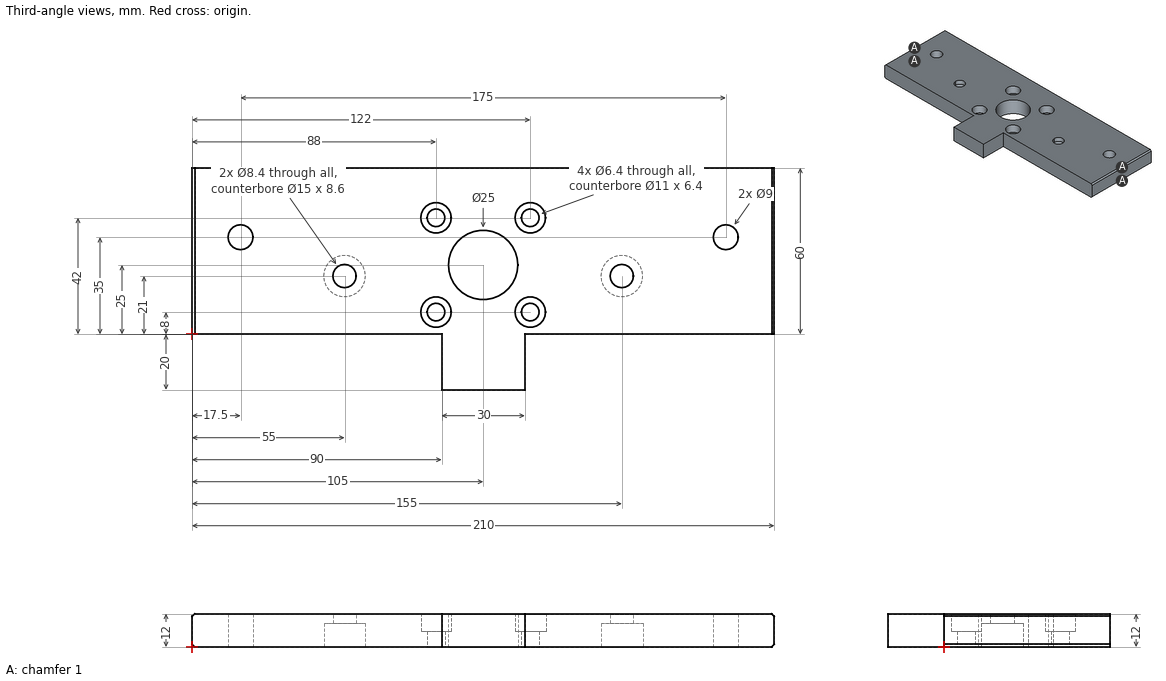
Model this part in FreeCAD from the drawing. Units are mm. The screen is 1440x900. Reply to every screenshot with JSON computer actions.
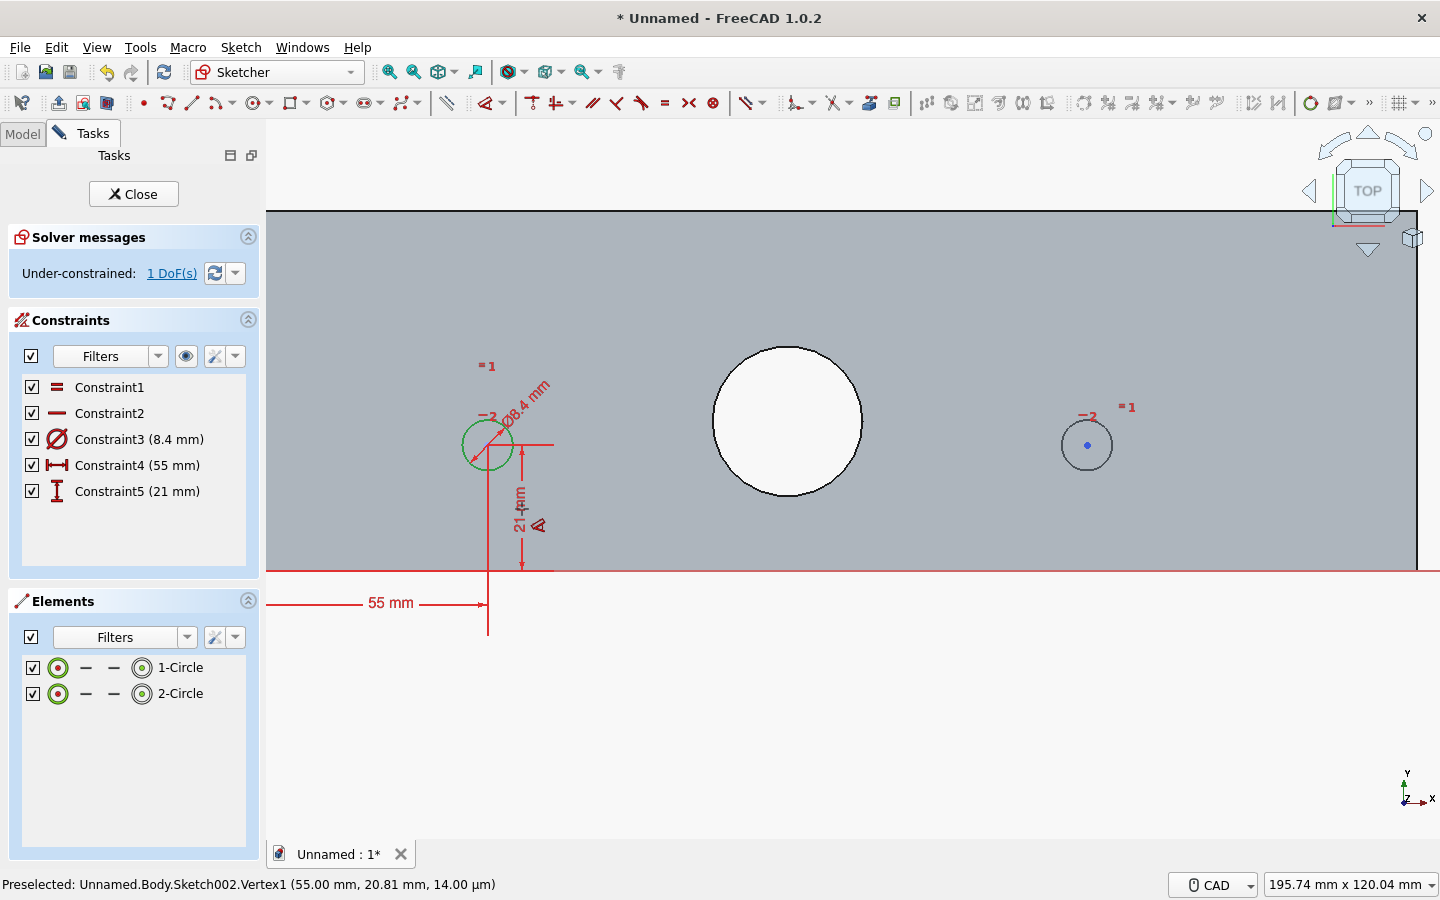
{"action": "left_click", "coordinate": [1087, 445]}
{"action": "left_click", "coordinate": [691, 605]}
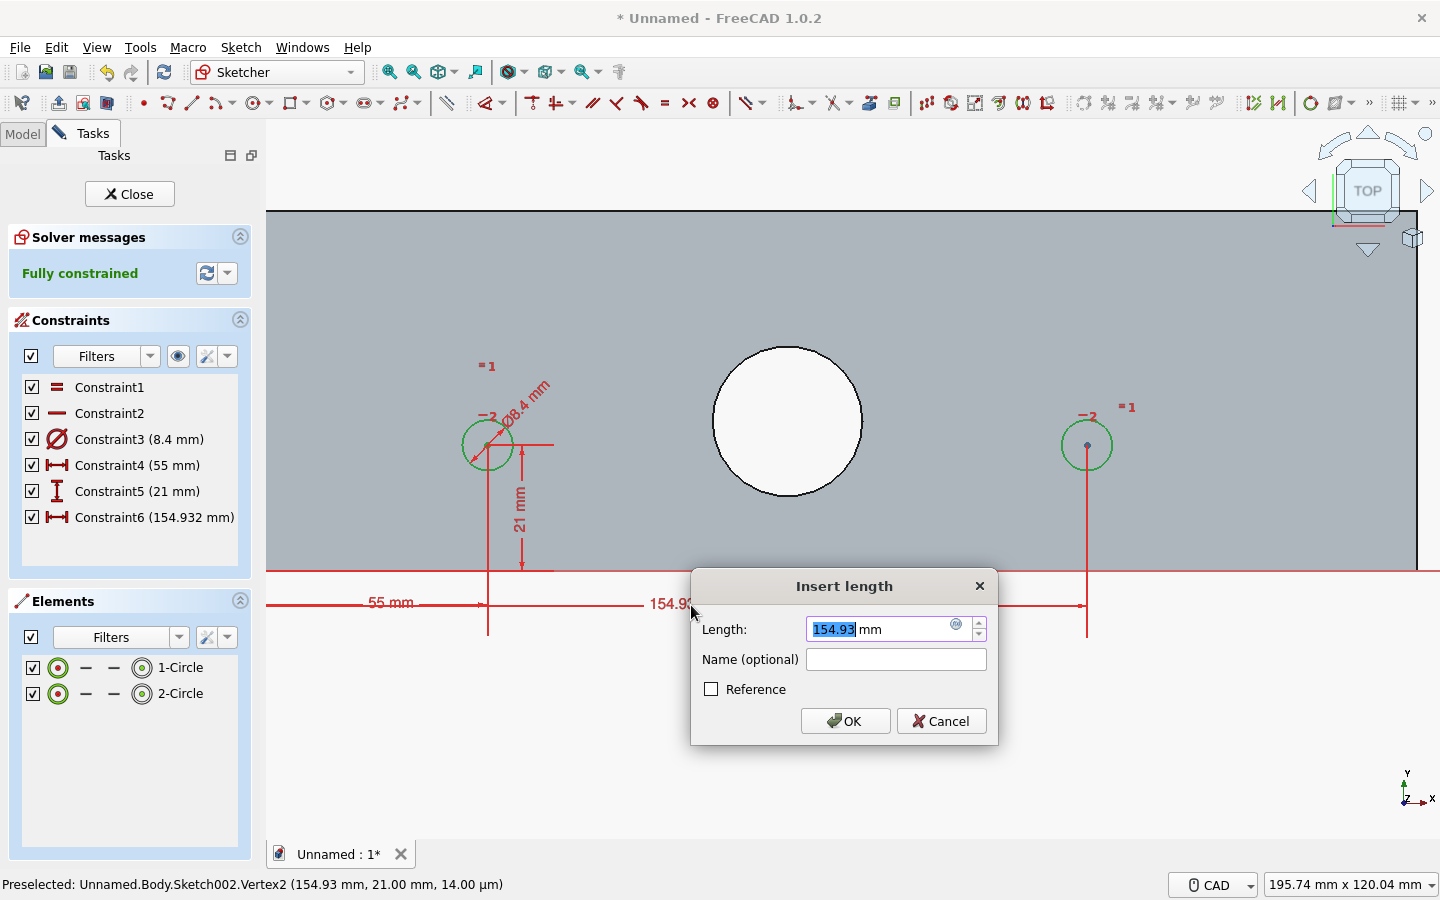
{"action": "type", "text": "155"}
{"action": "key", "text": "Return"}
{"action": "key", "text": "Escape"}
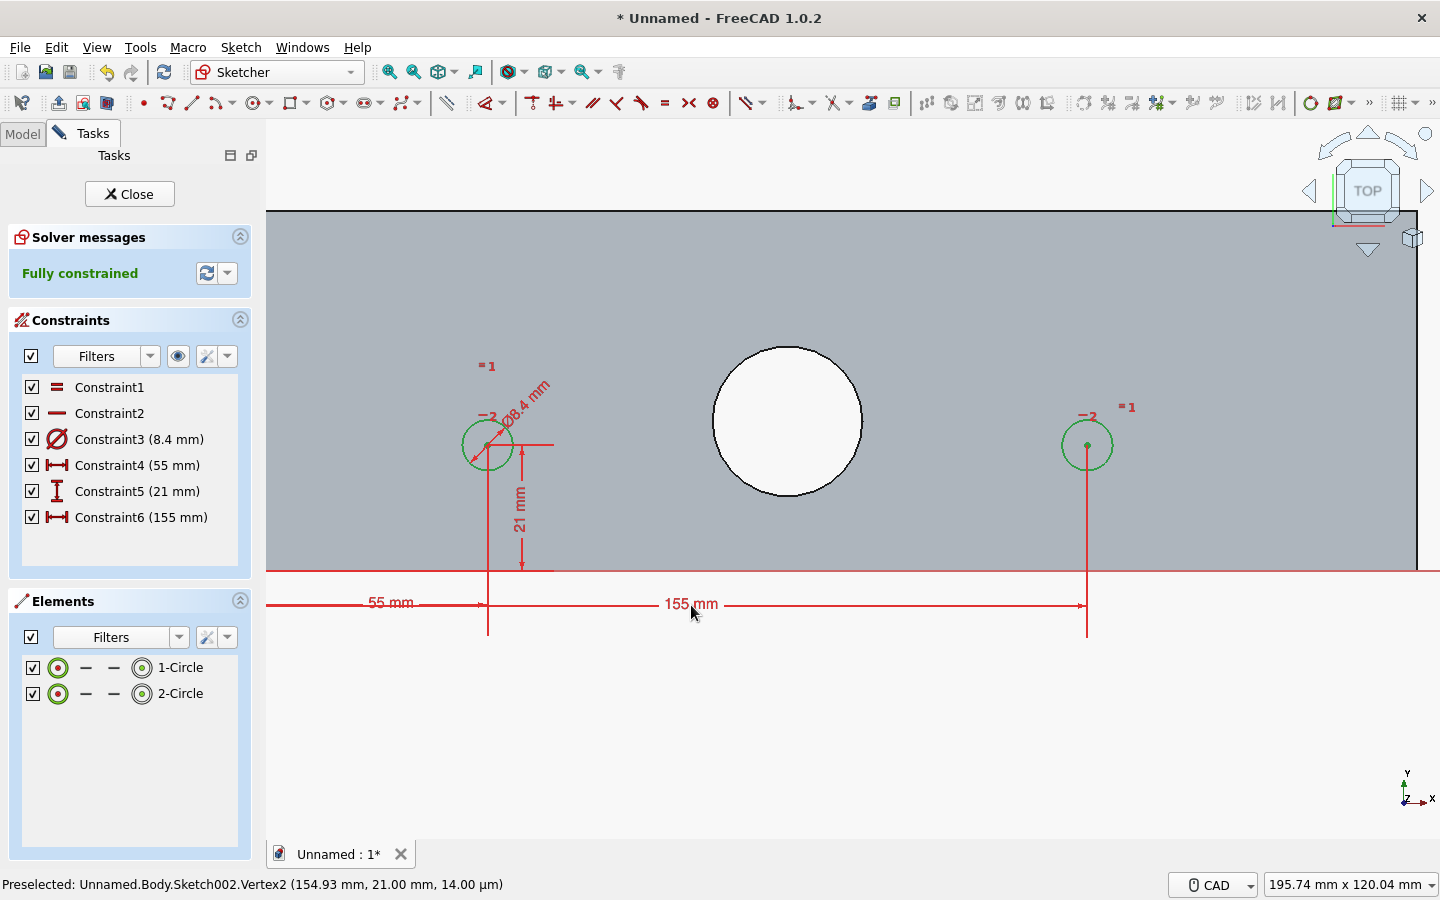
{"action": "left_click", "coordinate": [130, 194]}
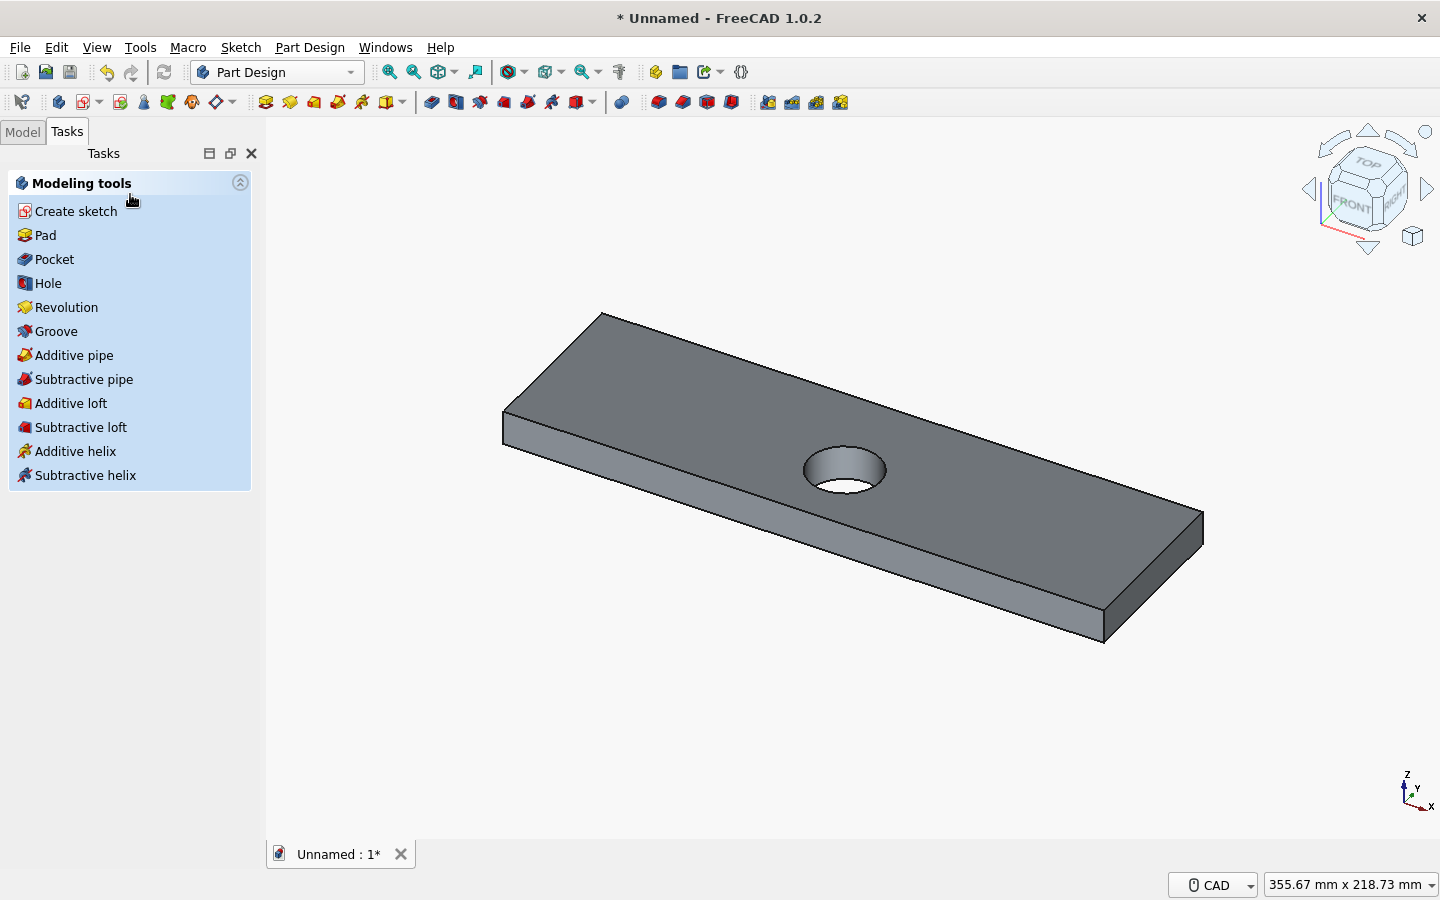
{"action": "left_click", "coordinate": [456, 102]}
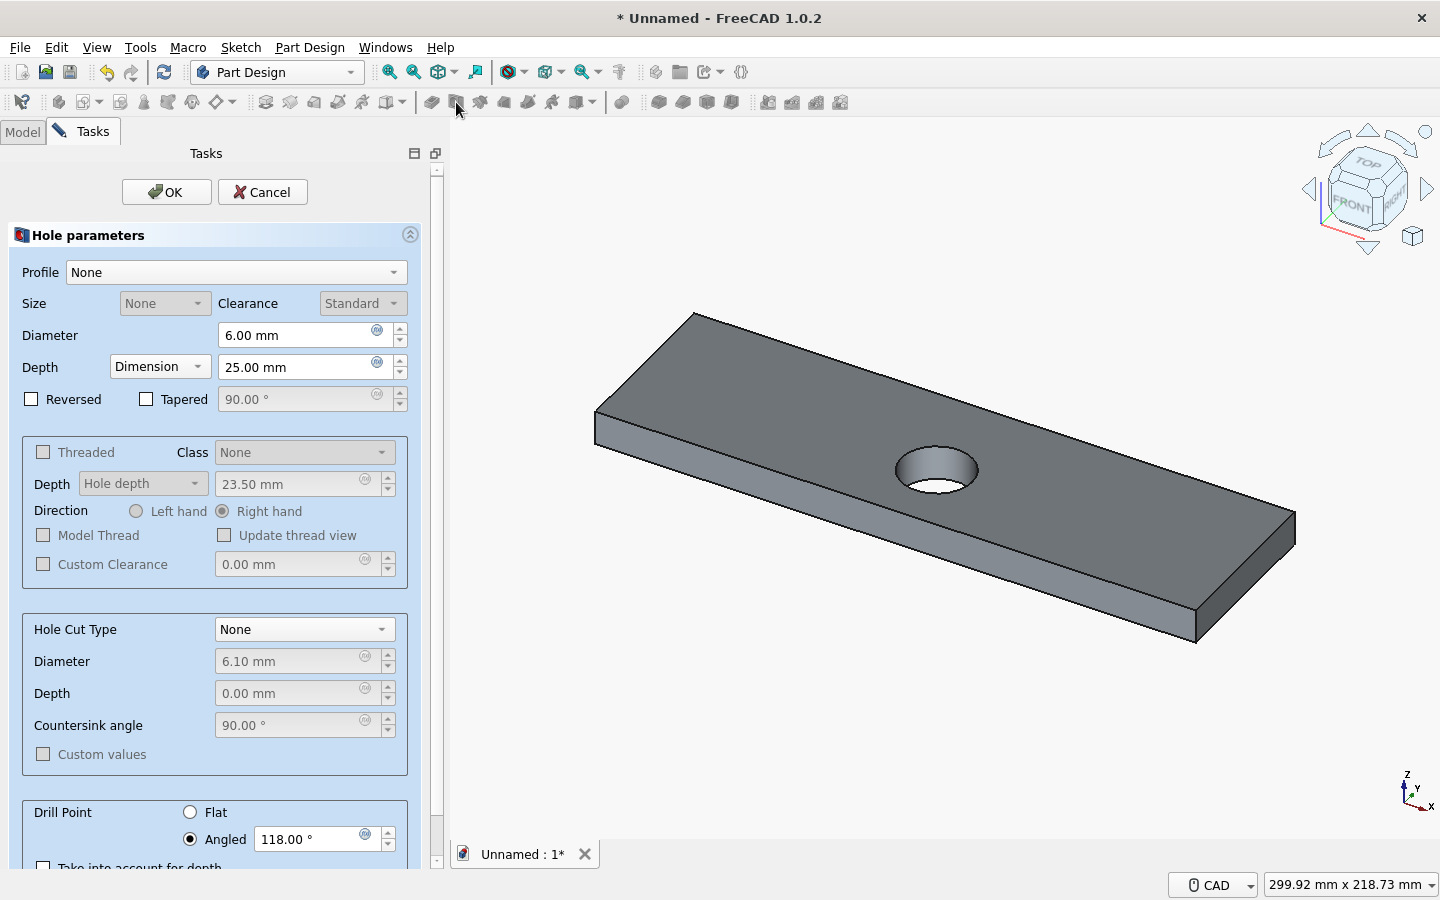
{"action": "triple_click", "coordinate": [305, 335]}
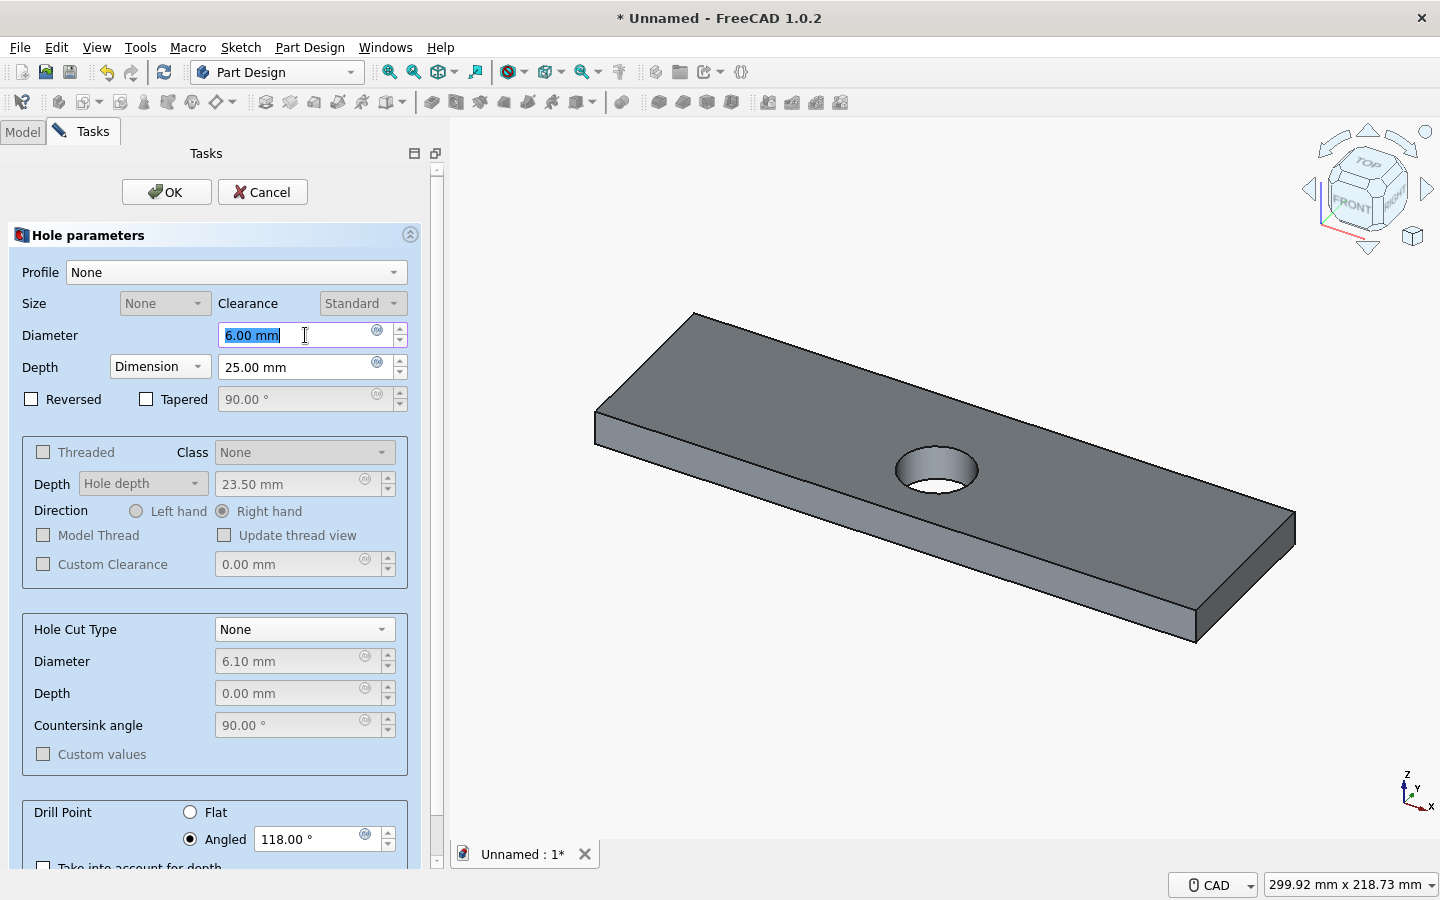
{"action": "type", "text": "8.4"}
{"action": "key", "text": "Tab"}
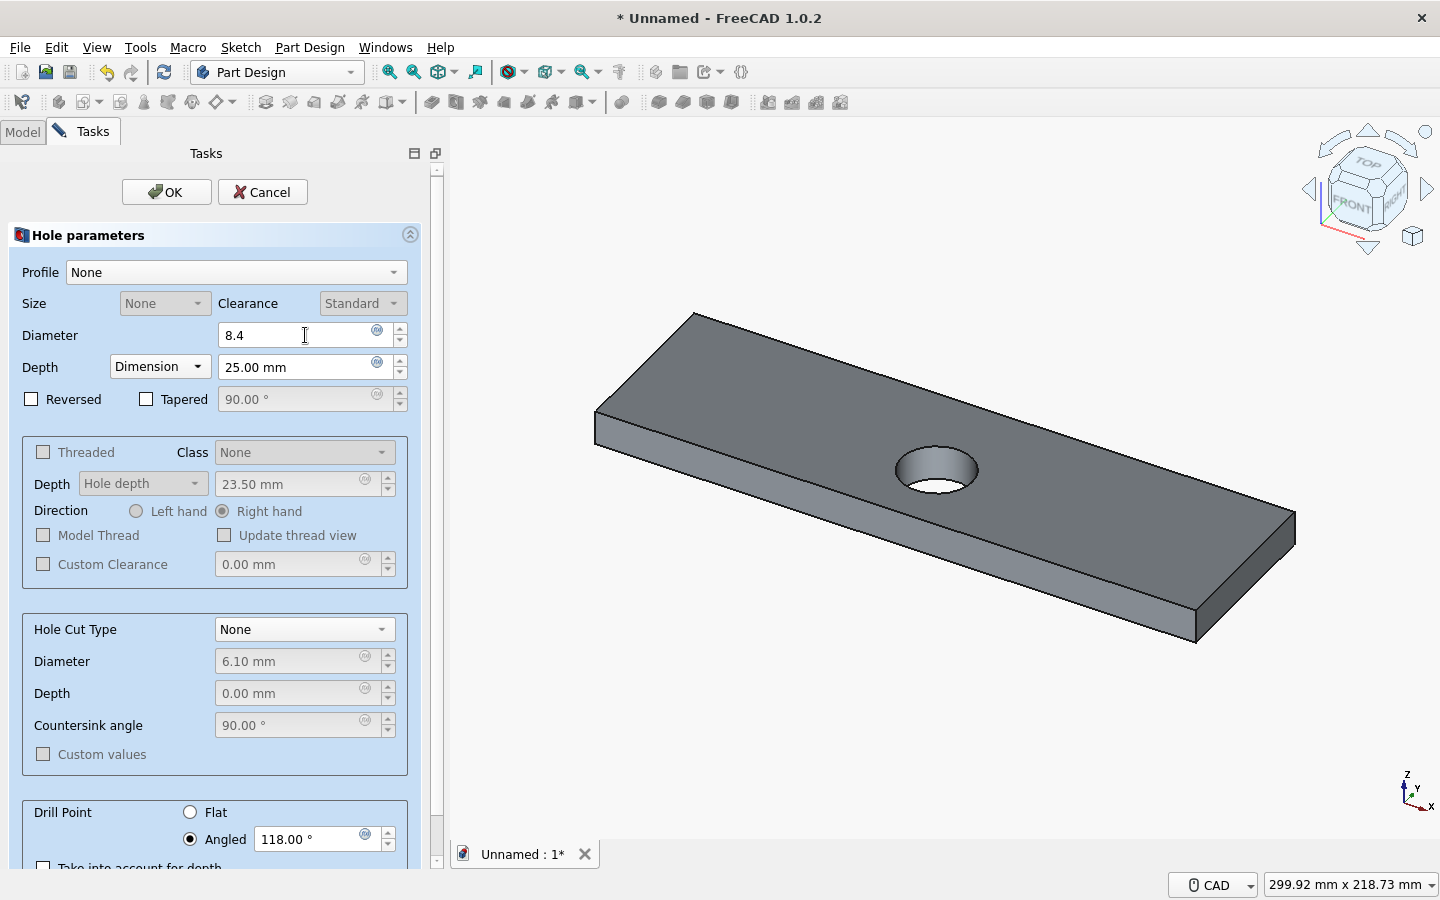
{"action": "left_click", "coordinate": [161, 366]}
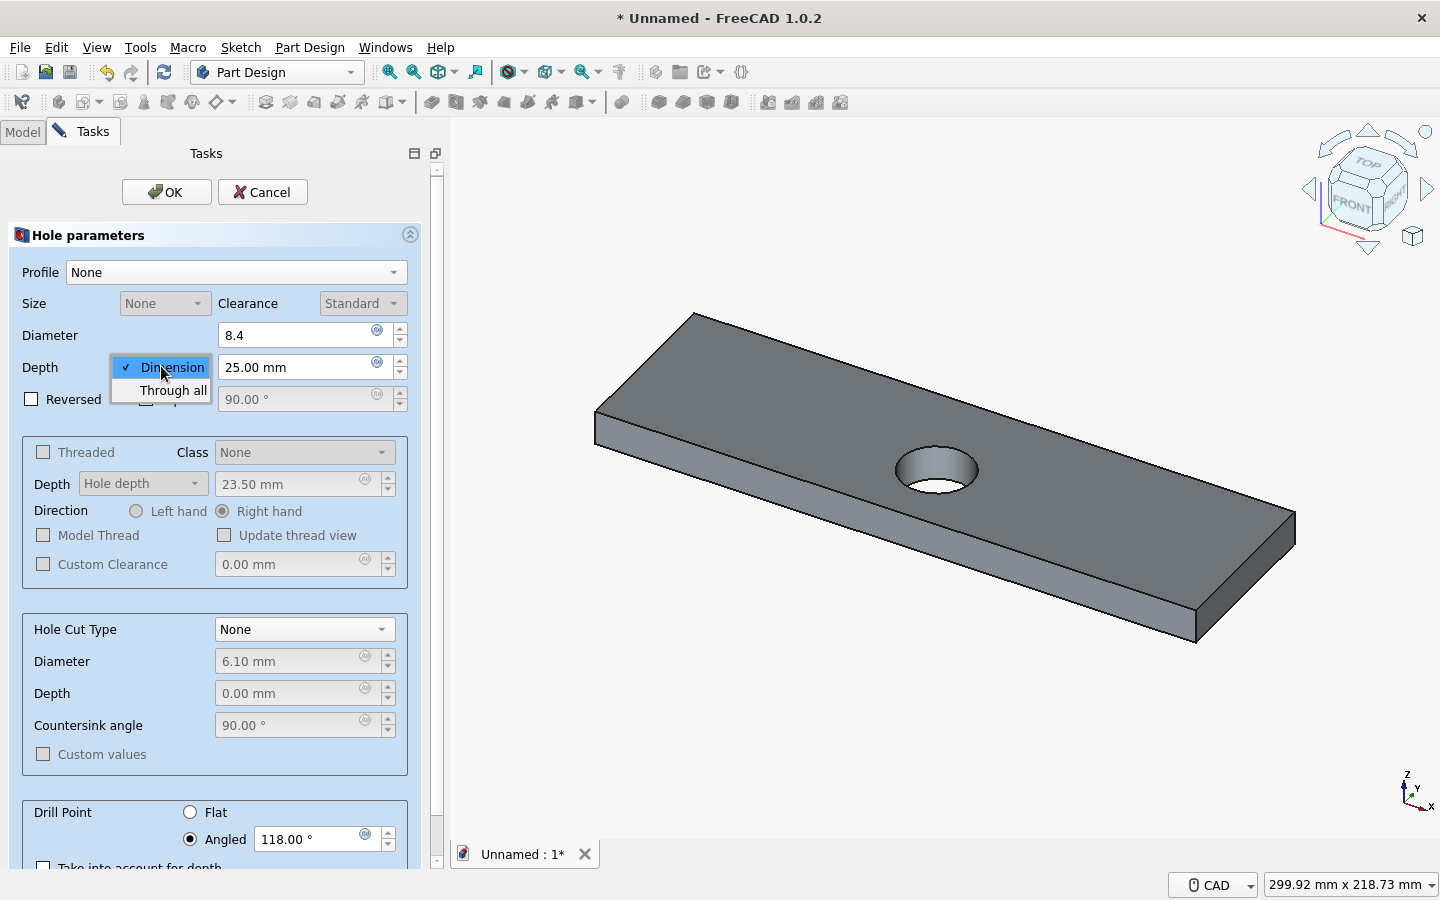
{"action": "left_click", "coordinate": [160, 390]}